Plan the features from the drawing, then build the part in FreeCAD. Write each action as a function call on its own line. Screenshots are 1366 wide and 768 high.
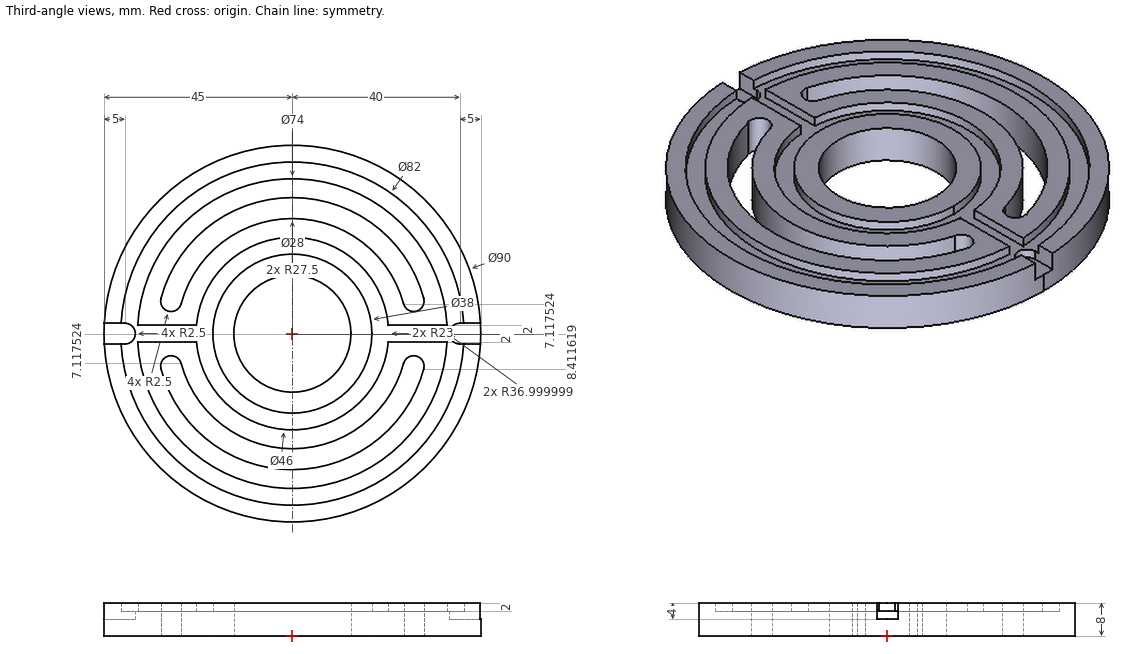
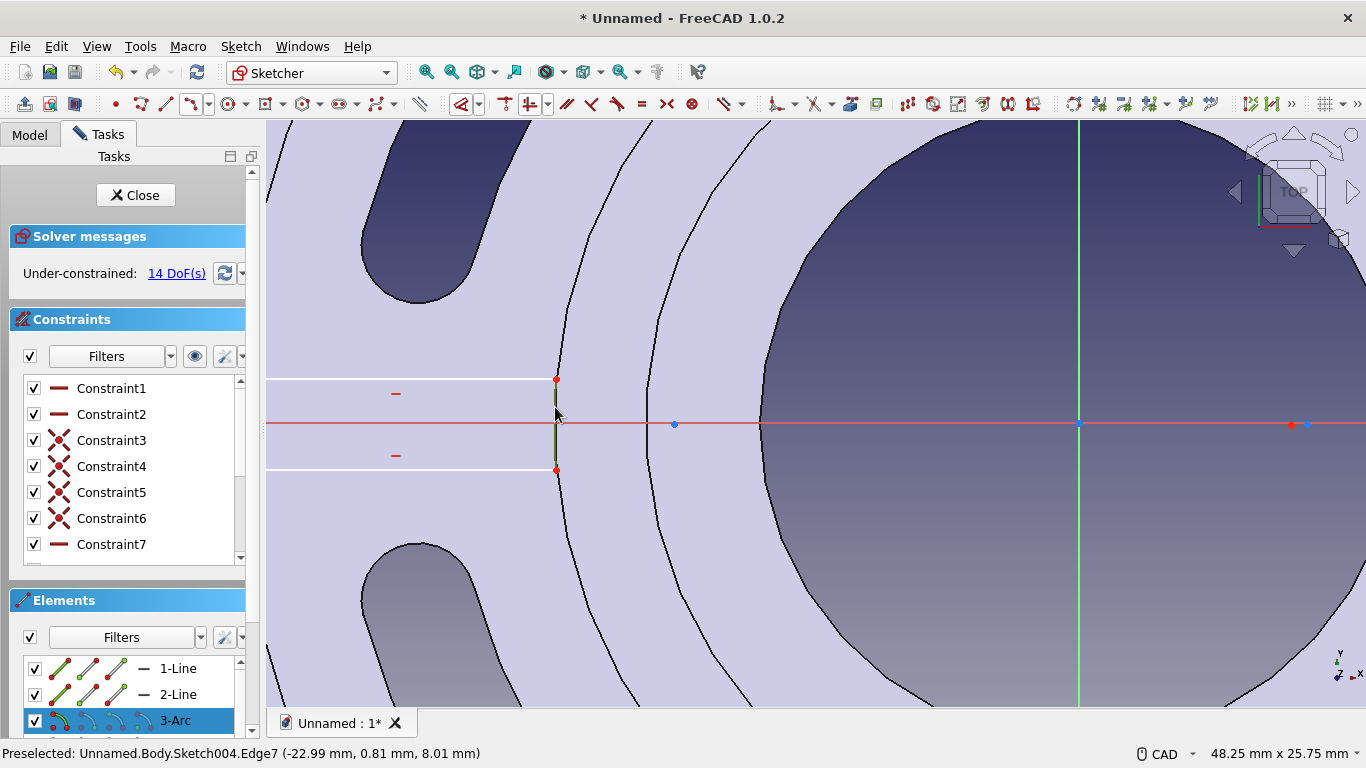
click(505, 104)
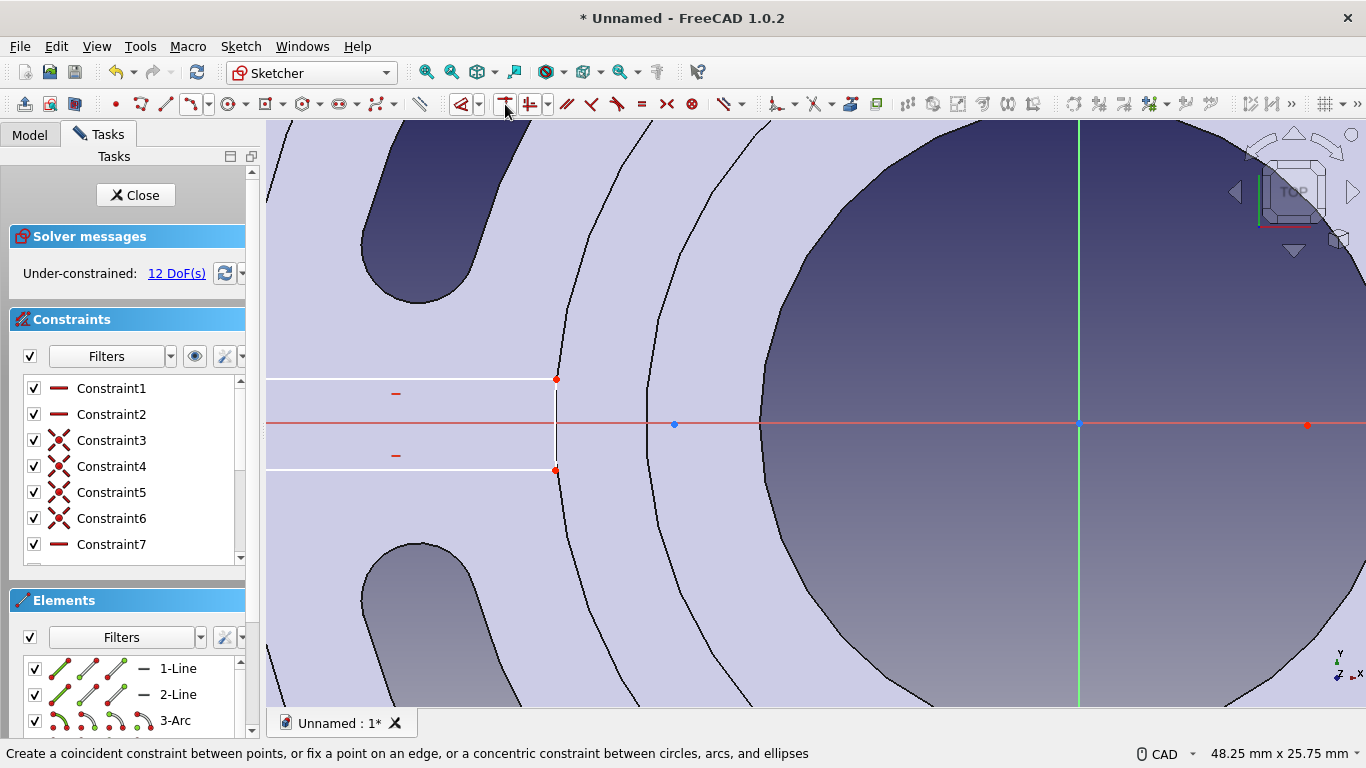
scroll(555, 408, down, 5)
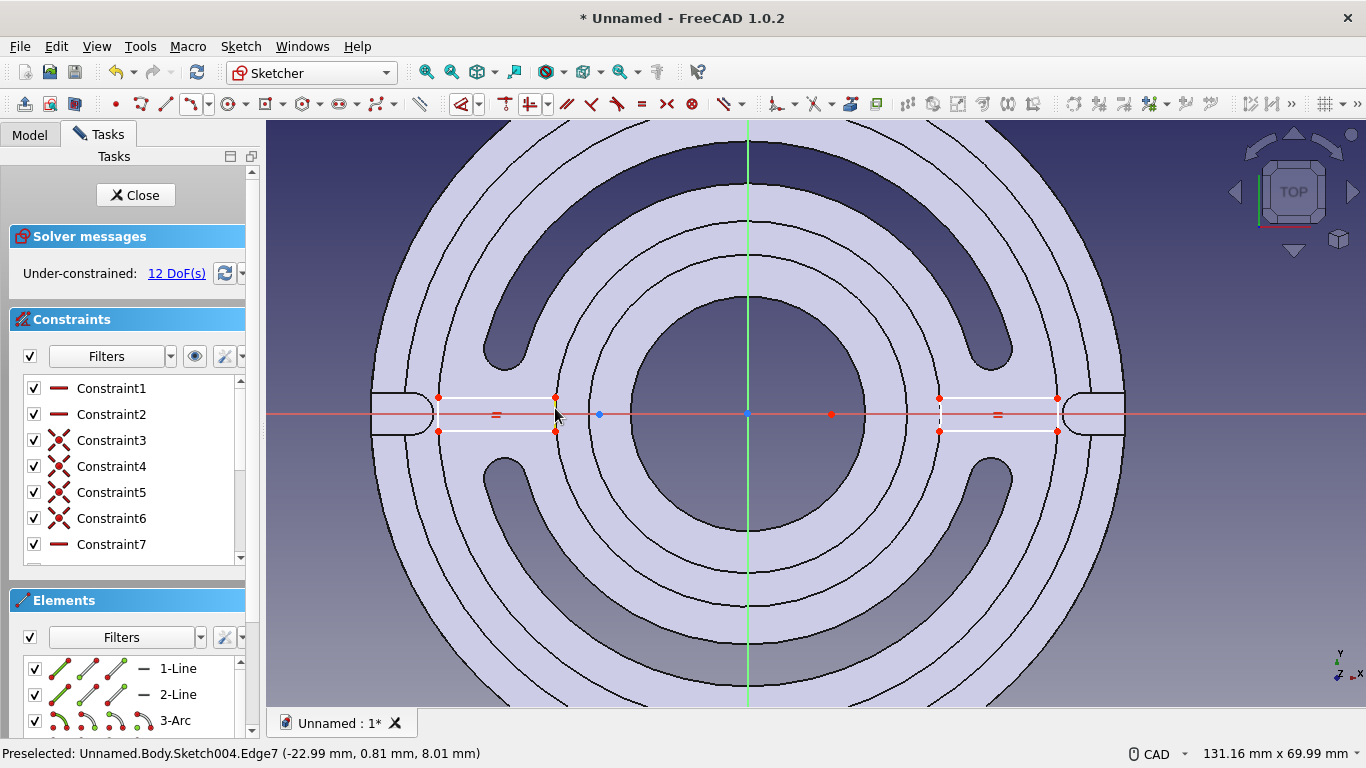
scroll(1058, 421, up, 4)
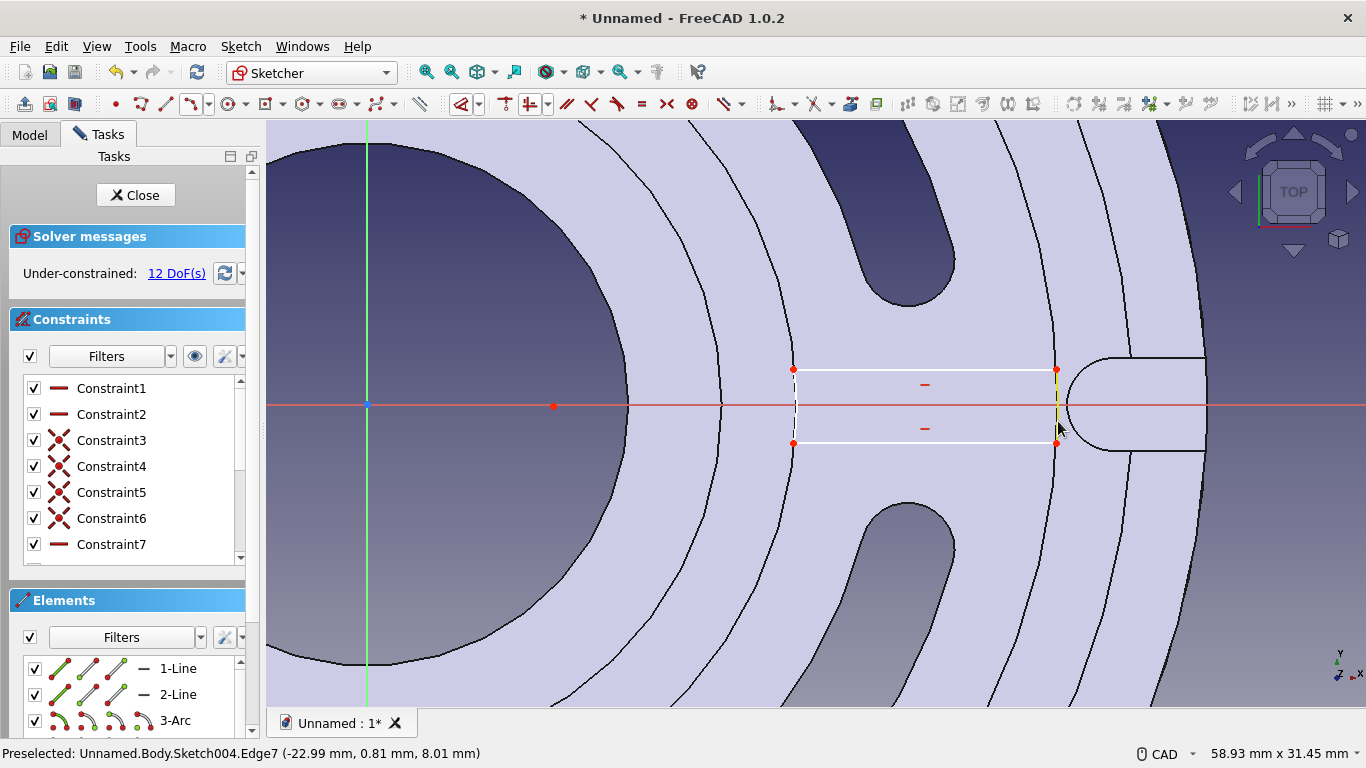
click(1058, 421)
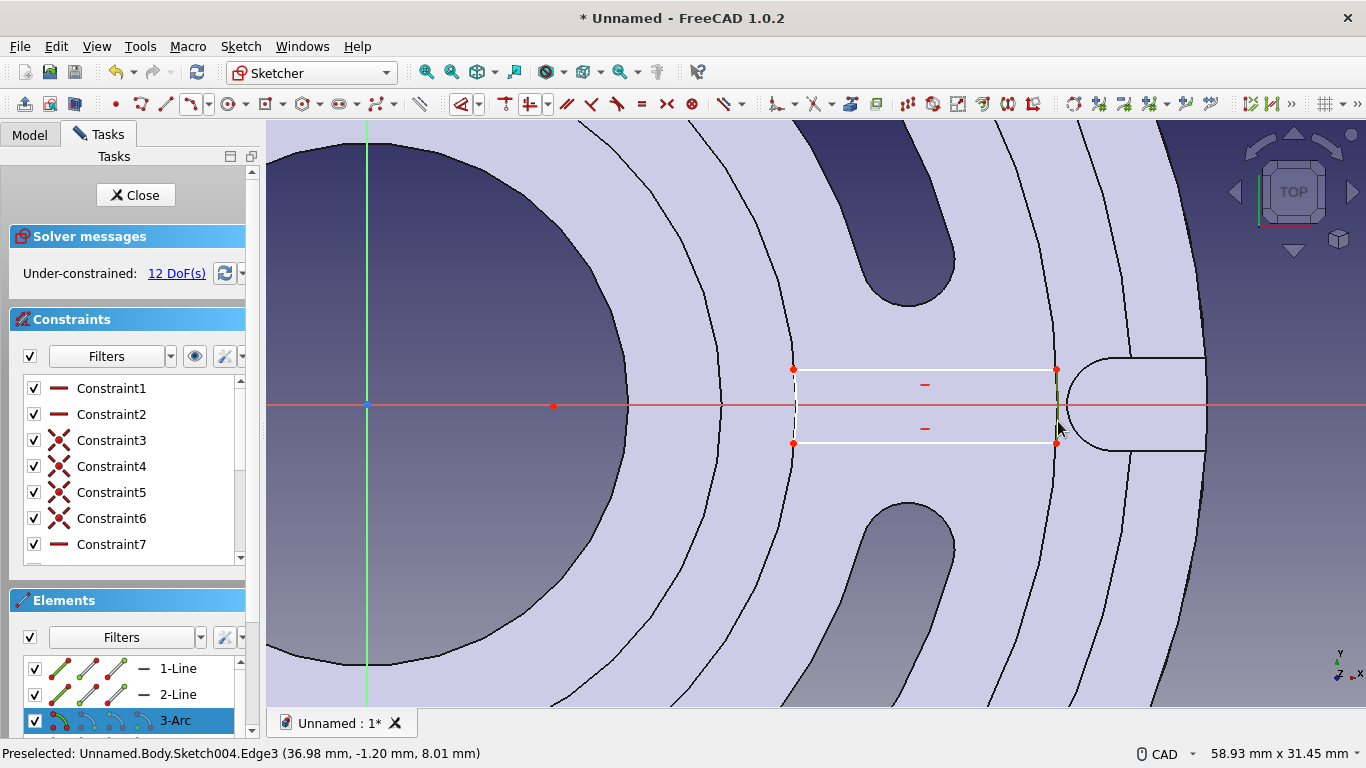
scroll(1058, 421, down, 4)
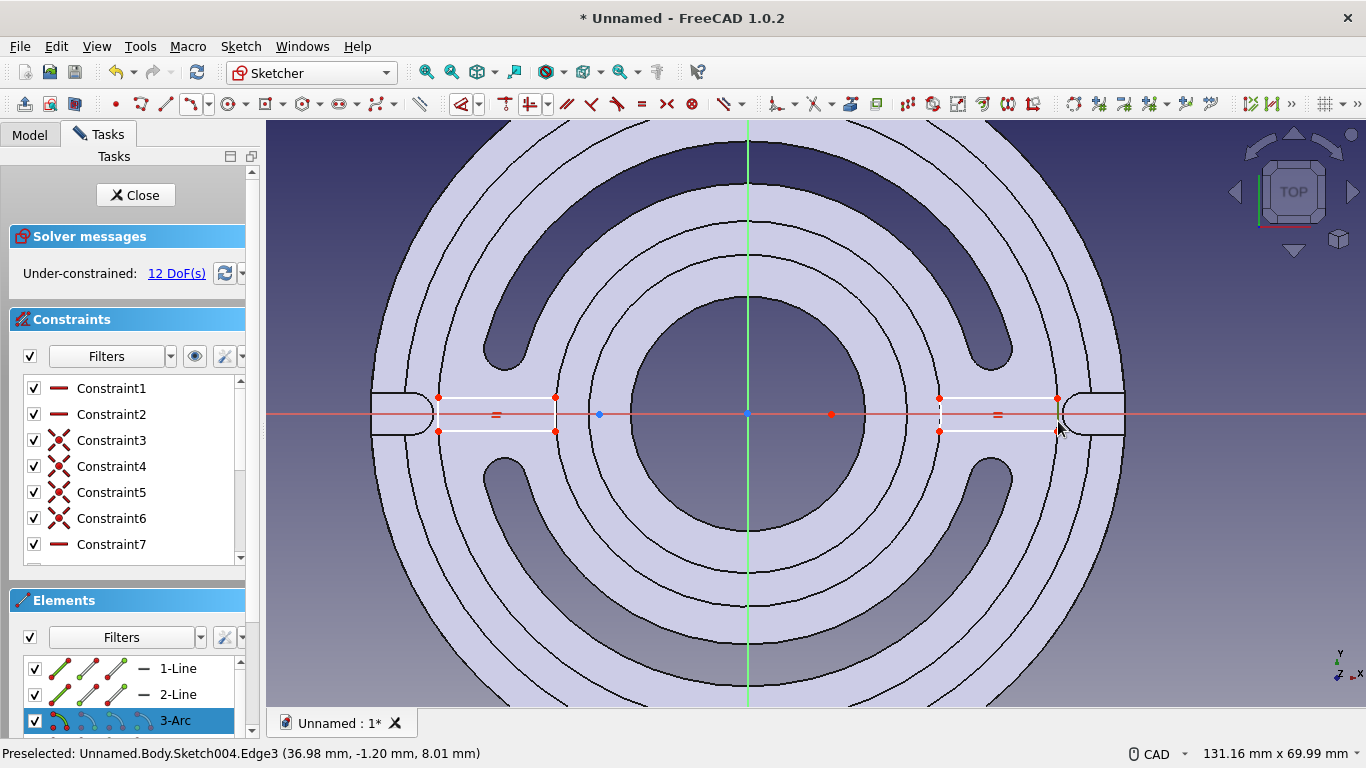
scroll(438, 408, up, 5)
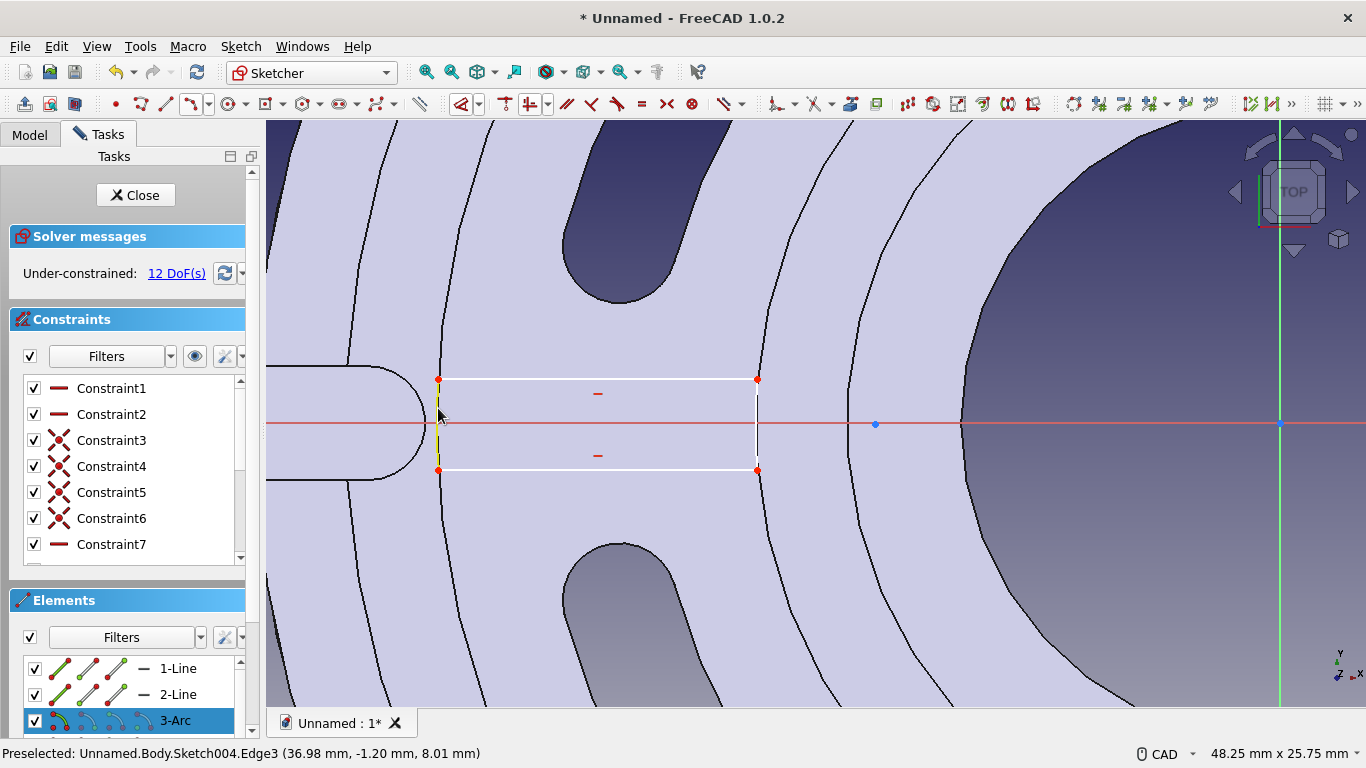
click(437, 406)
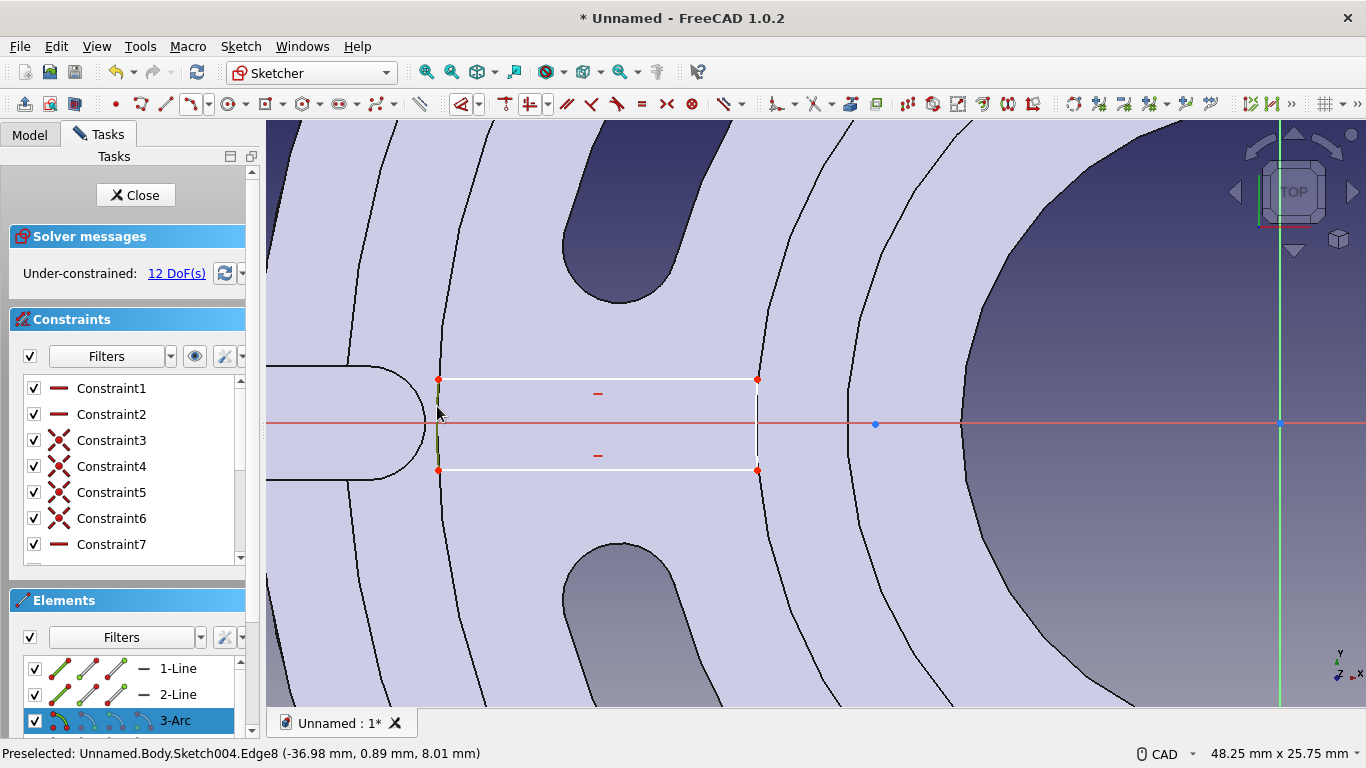
click(505, 104)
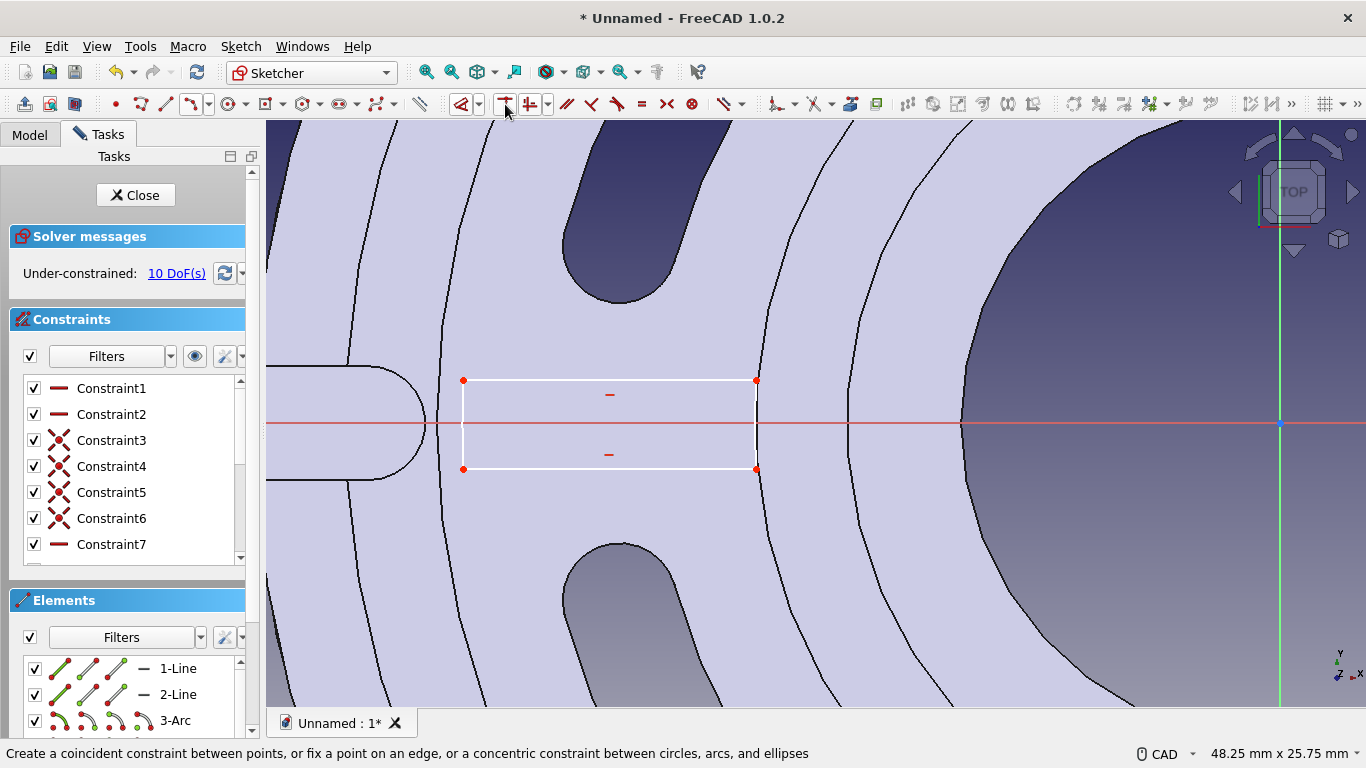
scroll(437, 408, down, 5)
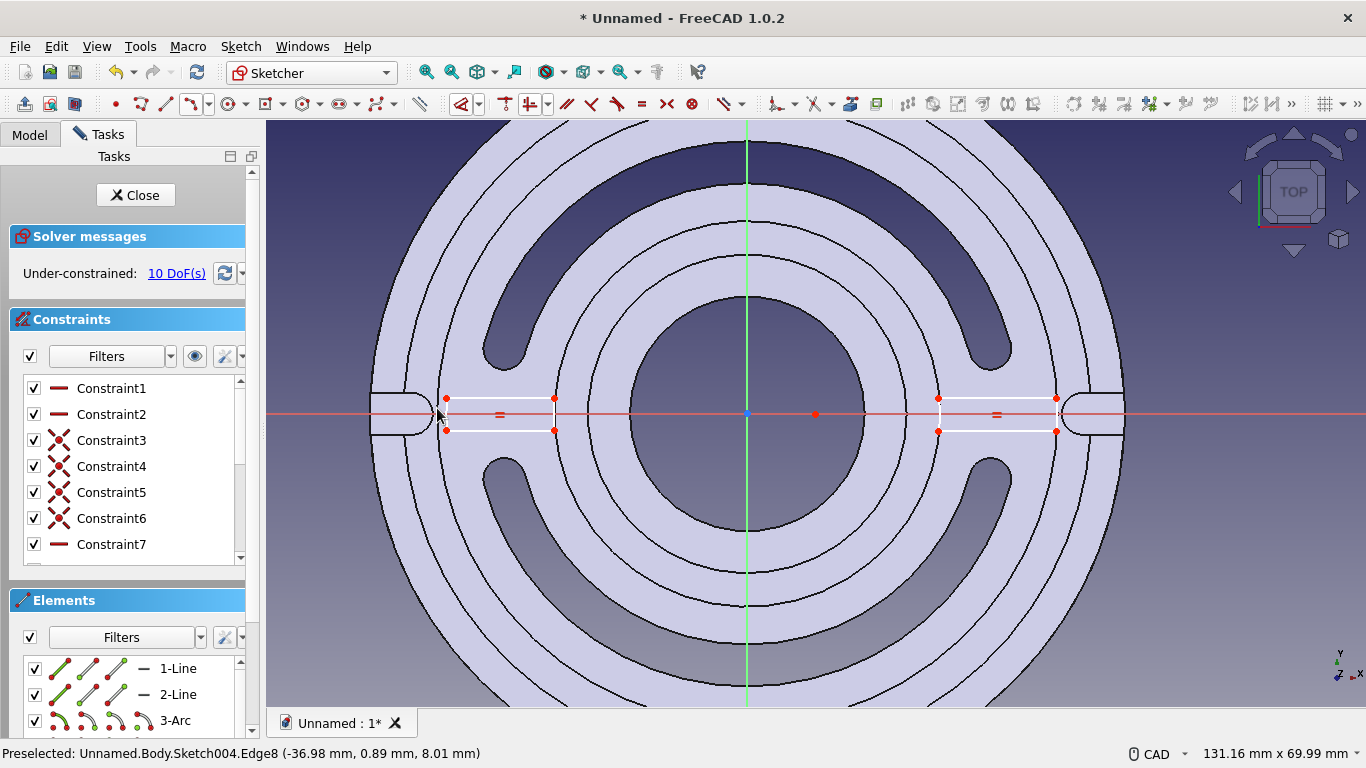
drag(737, 404, 825, 425)